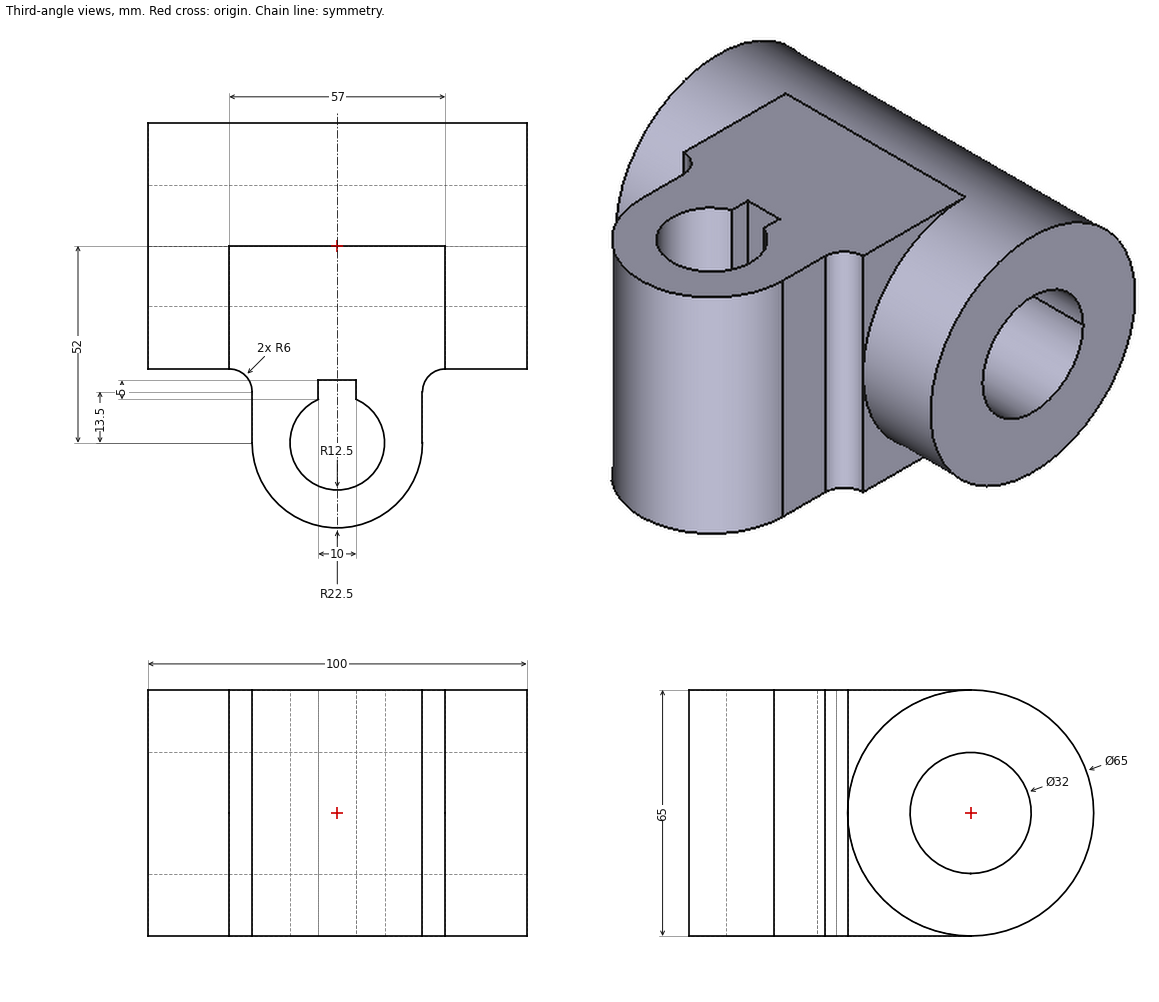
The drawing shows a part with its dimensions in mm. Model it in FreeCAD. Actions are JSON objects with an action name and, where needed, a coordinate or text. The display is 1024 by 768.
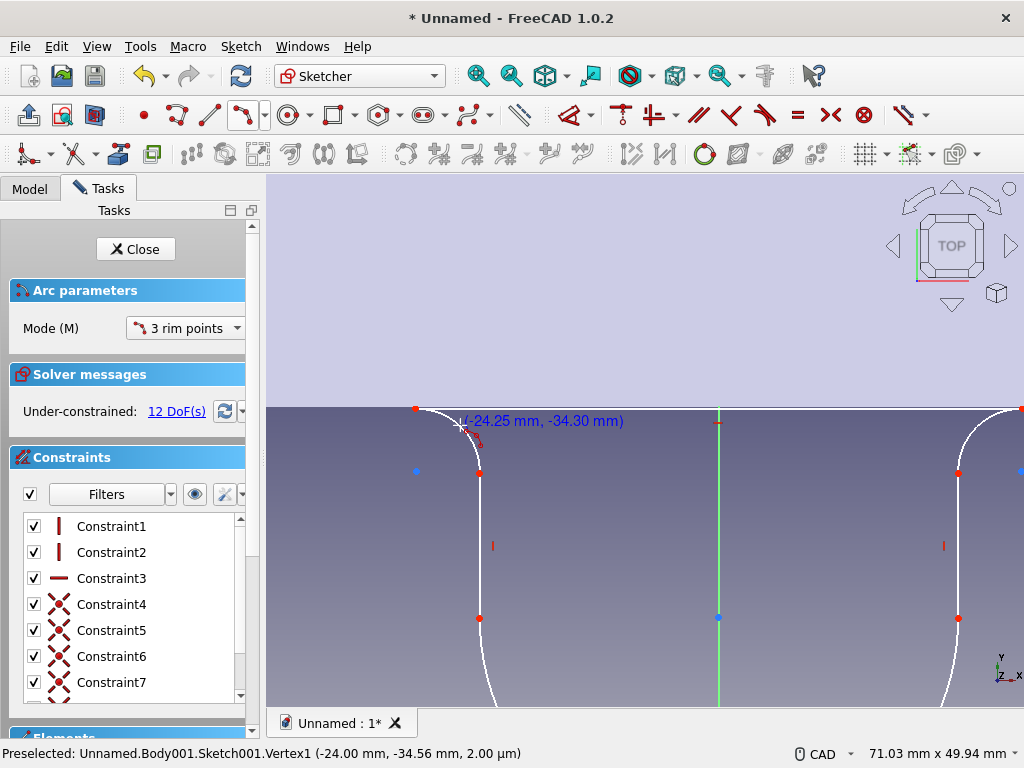
{"action": "left_click", "coordinate": [177, 116]}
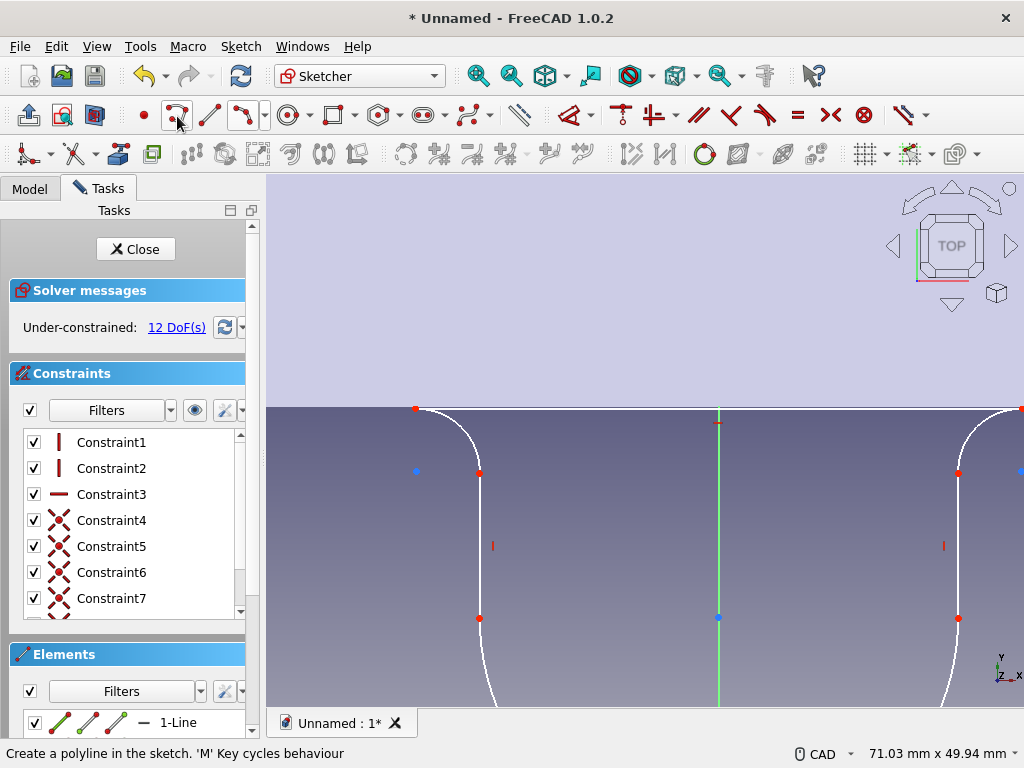
{"action": "left_click", "coordinate": [665, 493]}
{"action": "left_click", "coordinate": [665, 439]}
{"action": "left_click", "coordinate": [772, 439]}
{"action": "left_click", "coordinate": [772, 493]}
{"action": "right_click", "coordinate": [772, 493]}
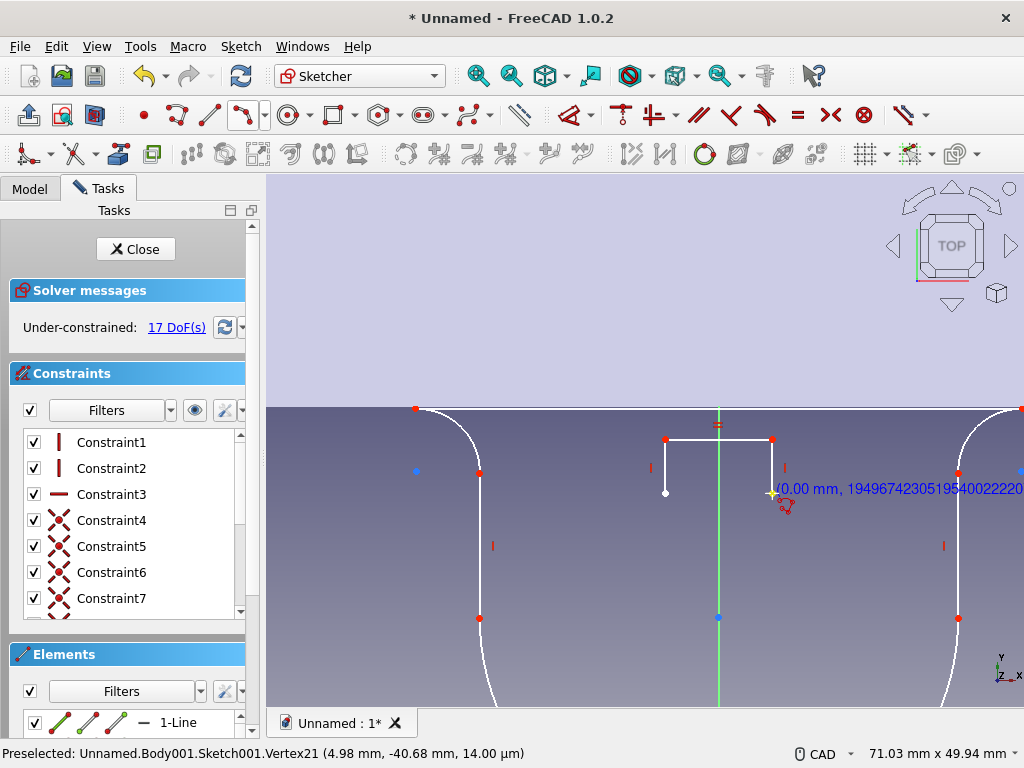
{"action": "key", "text": "g 3 a"}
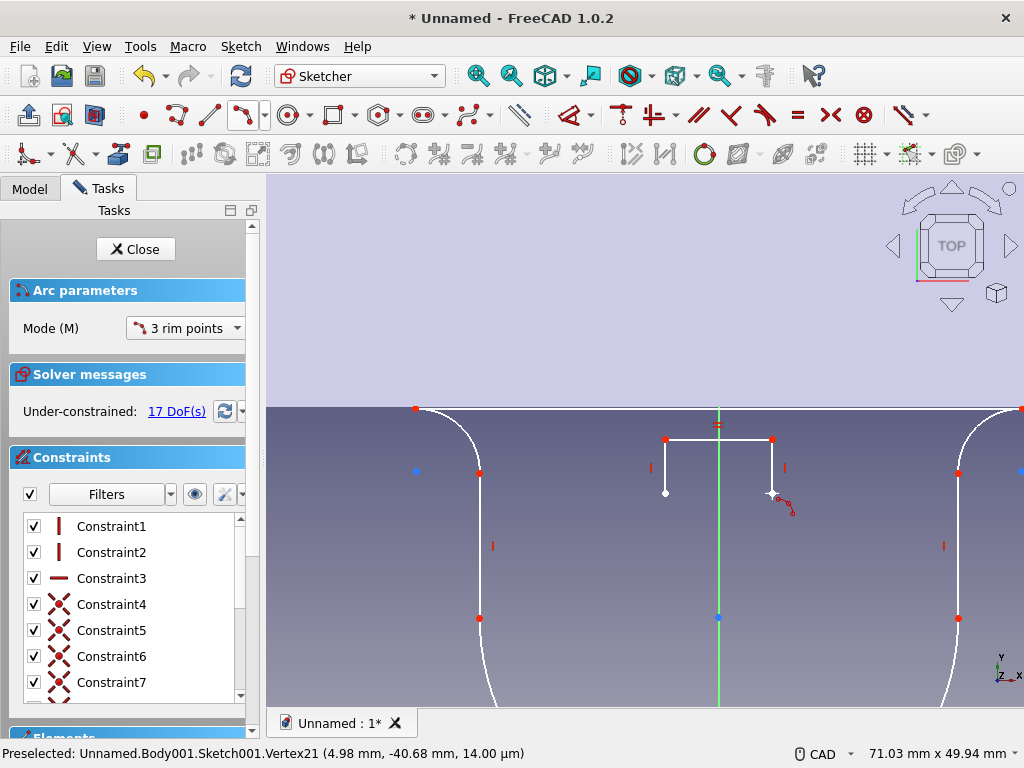
{"action": "left_click", "coordinate": [772, 494]}
{"action": "left_click", "coordinate": [665, 494]}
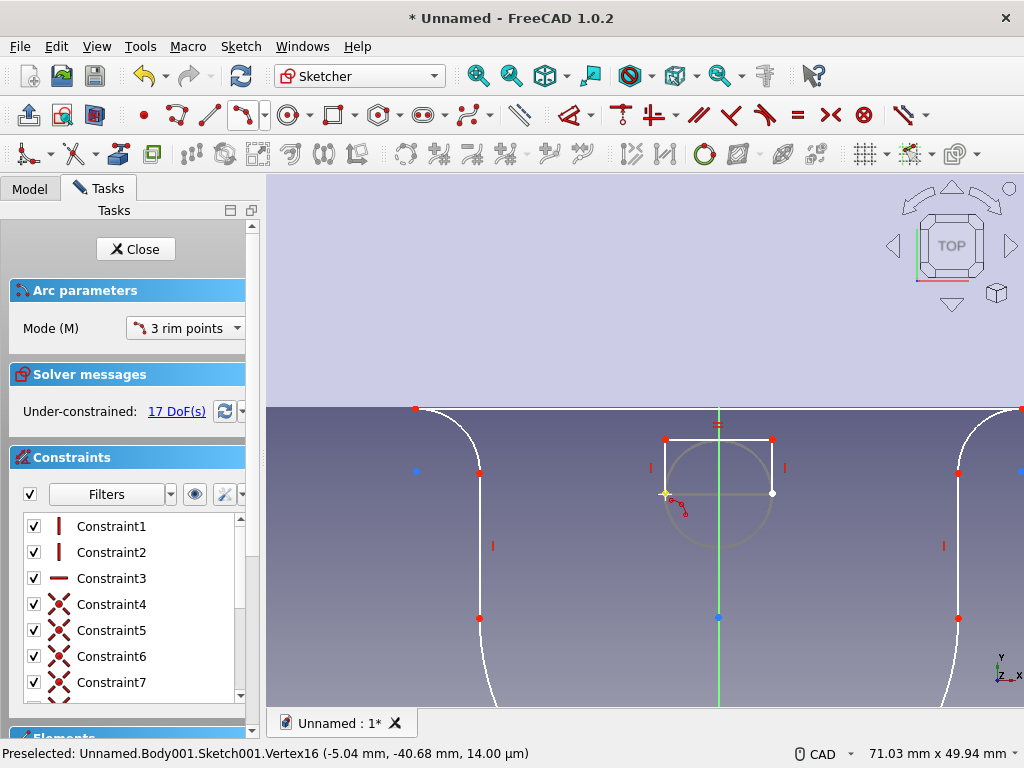
{"action": "scroll", "coordinate": [460, 427], "scroll_direction": "down", "scroll_amount": 4}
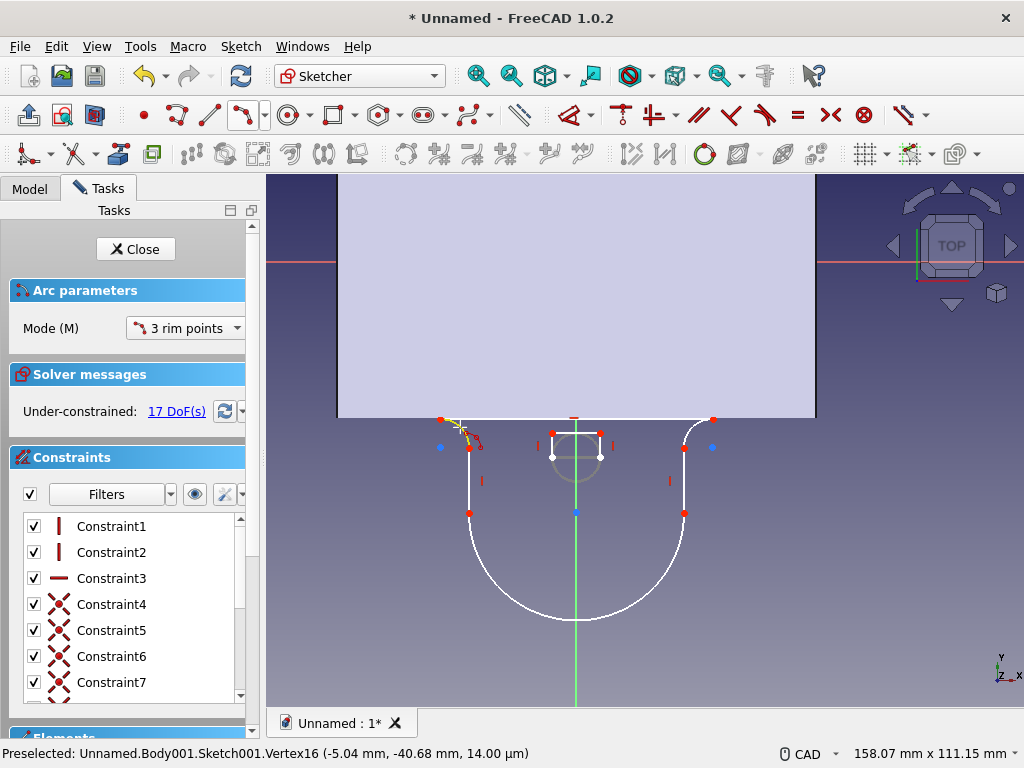
{"action": "left_click", "coordinate": [545, 563]}
{"action": "key", "text": "Escape"}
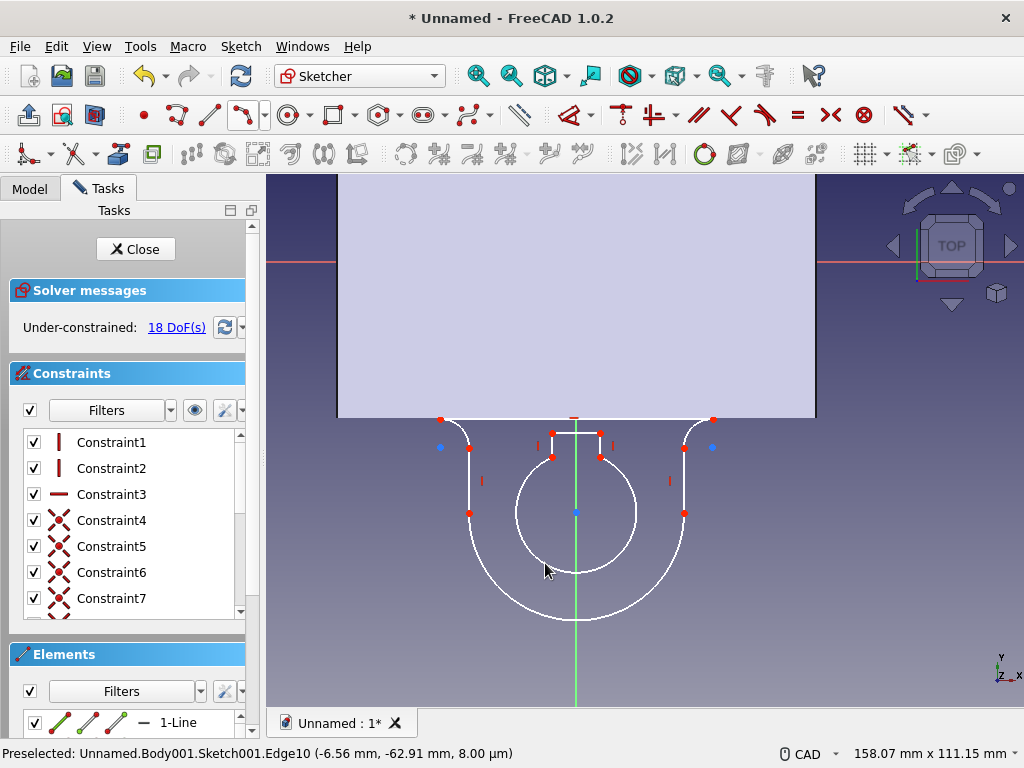
{"action": "left_click", "coordinate": [469, 468]}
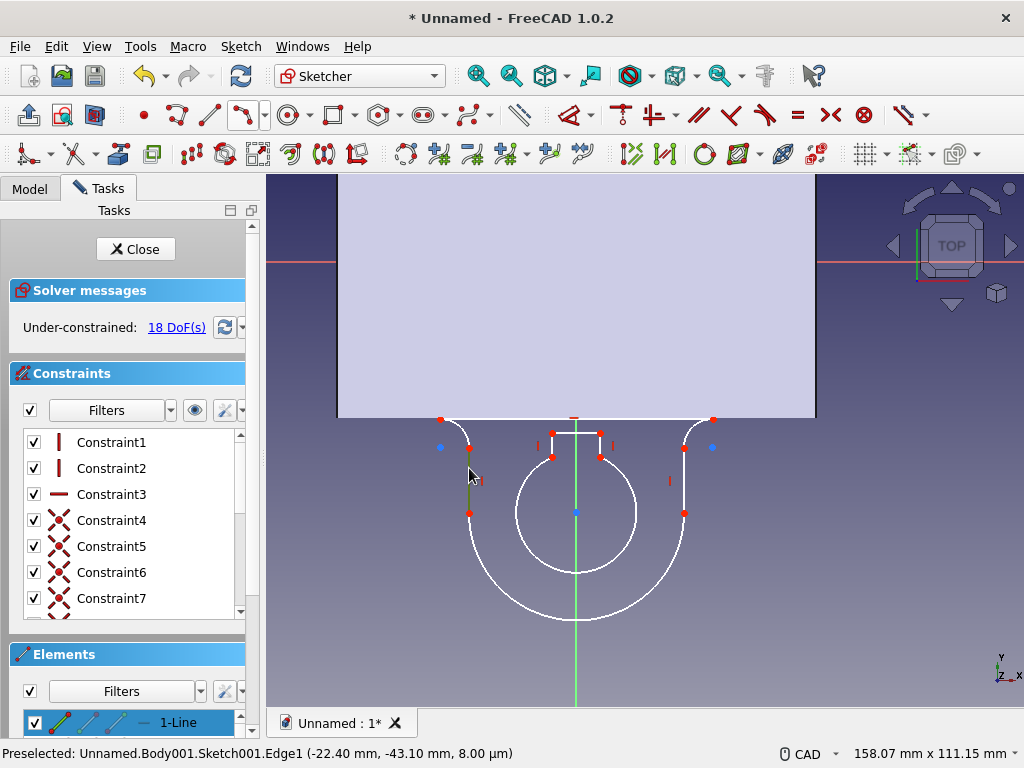
{"action": "left_click", "coordinate": [513, 600]}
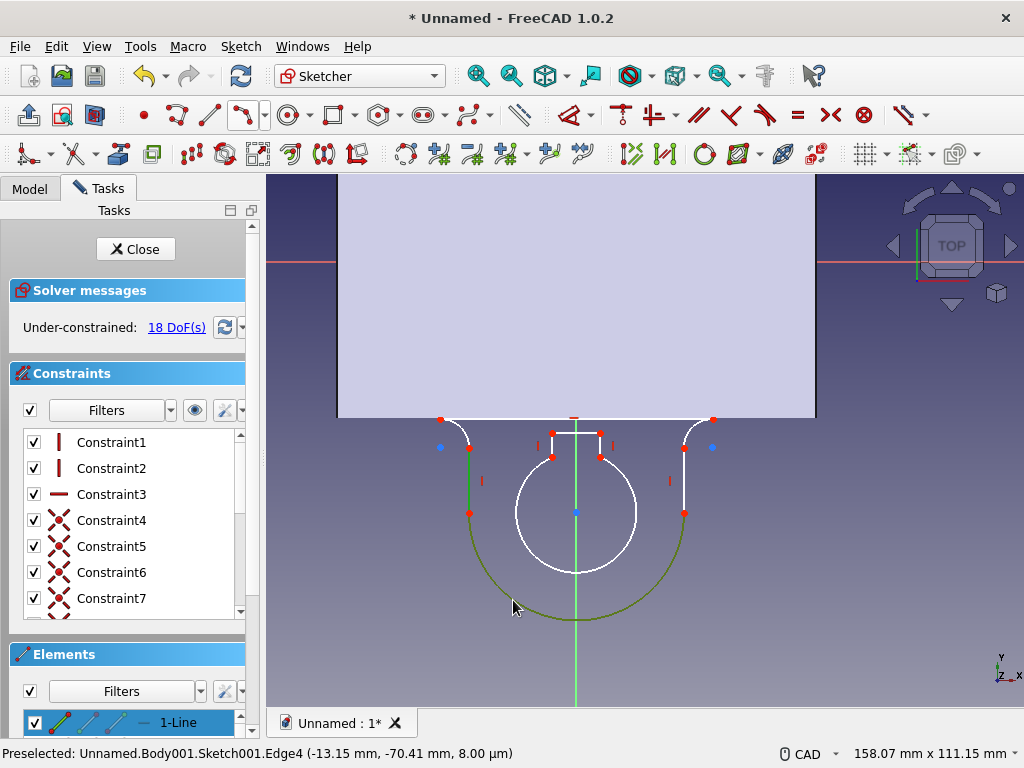
{"action": "left_click", "coordinate": [765, 116]}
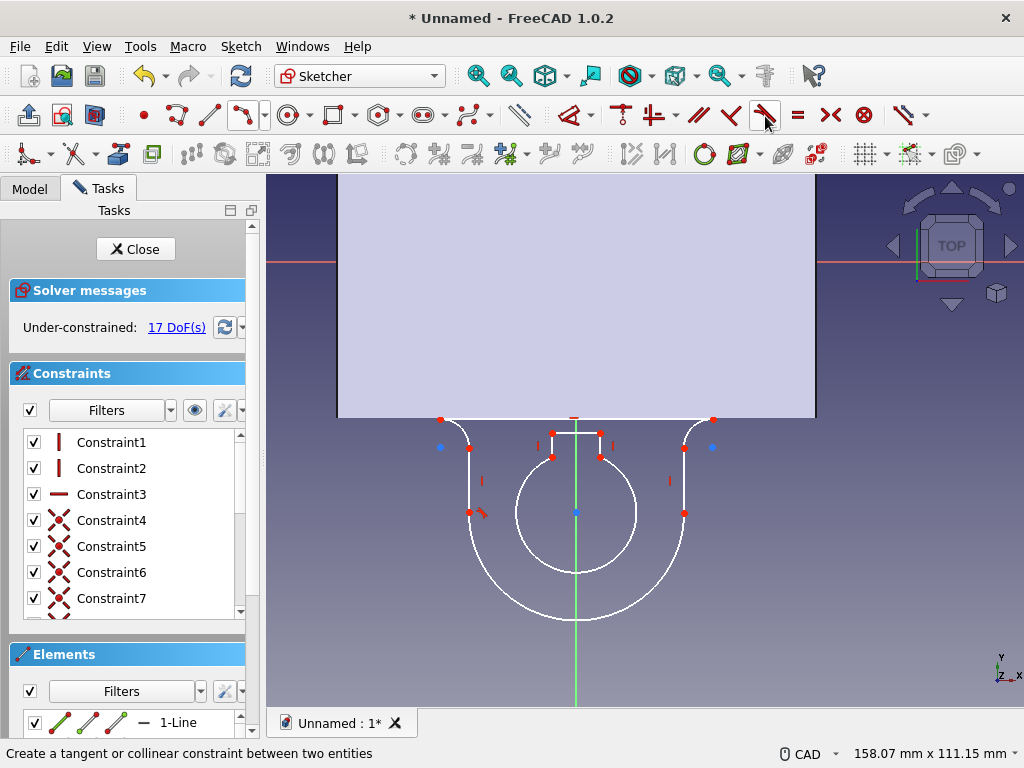
{"action": "left_click", "coordinate": [469, 468]}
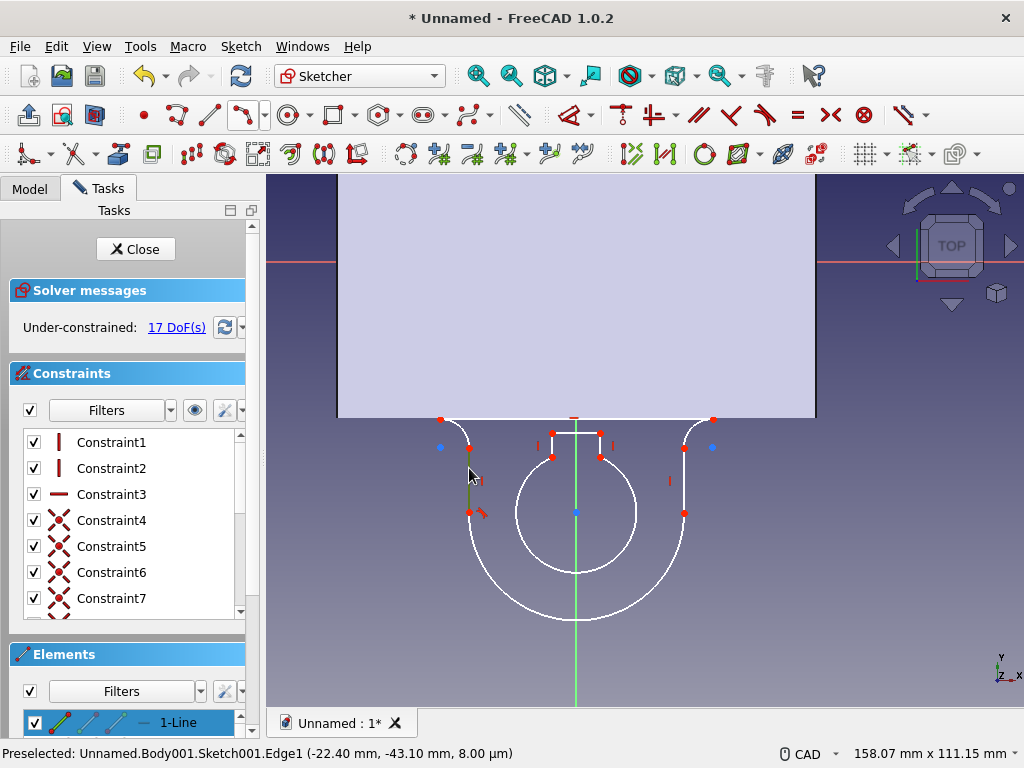
{"action": "left_click", "coordinate": [466, 435]}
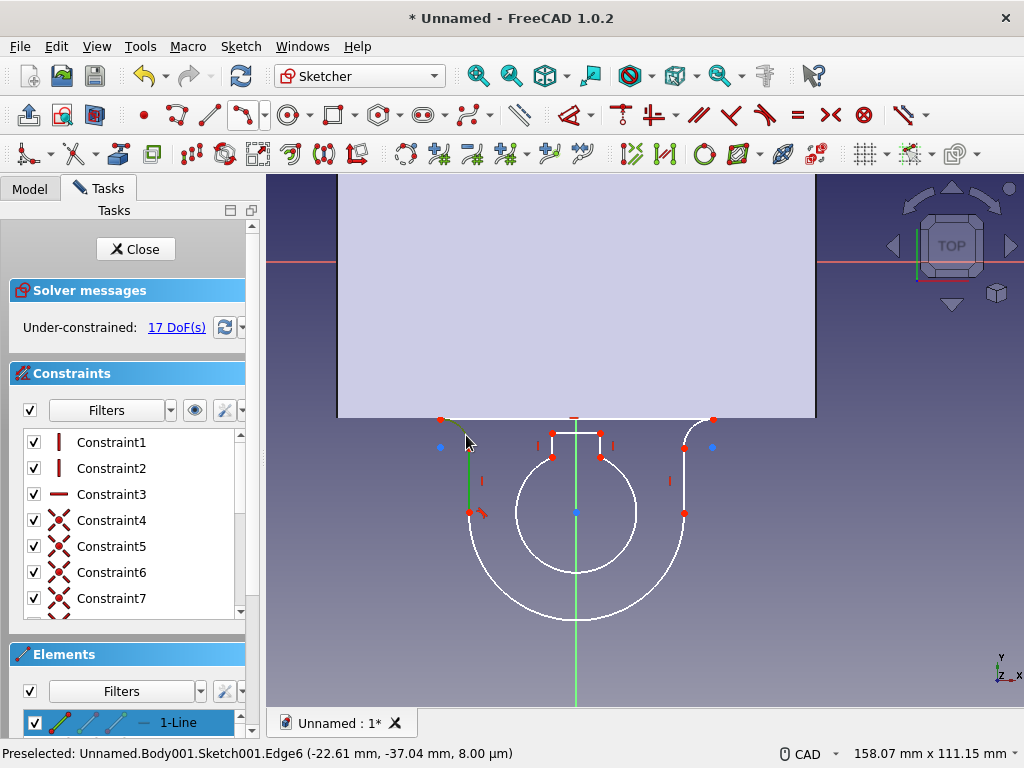
{"action": "key", "text": "t"}